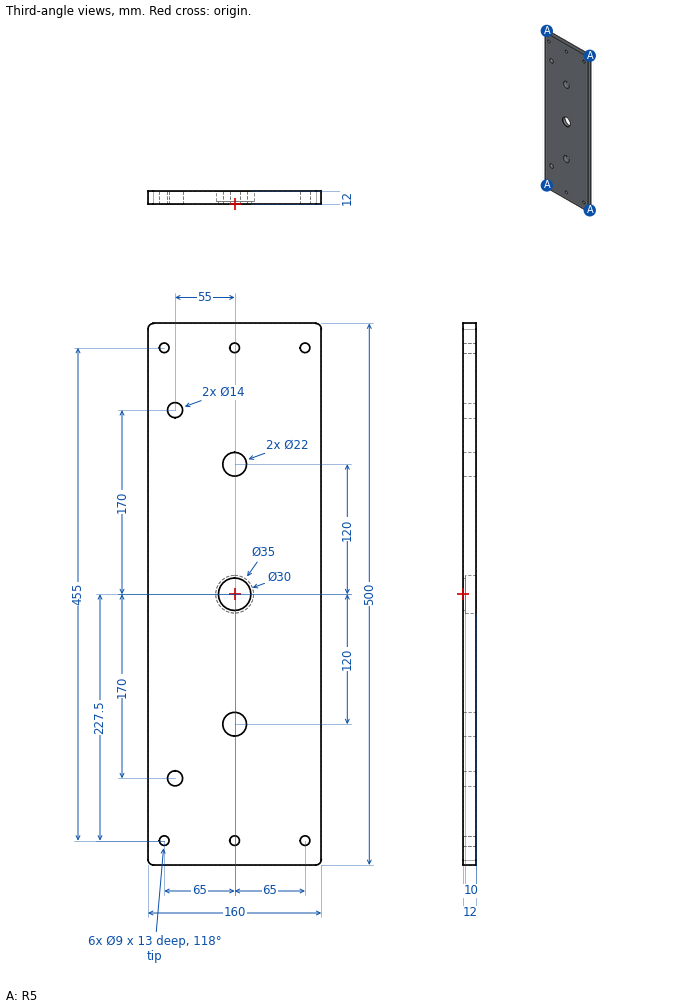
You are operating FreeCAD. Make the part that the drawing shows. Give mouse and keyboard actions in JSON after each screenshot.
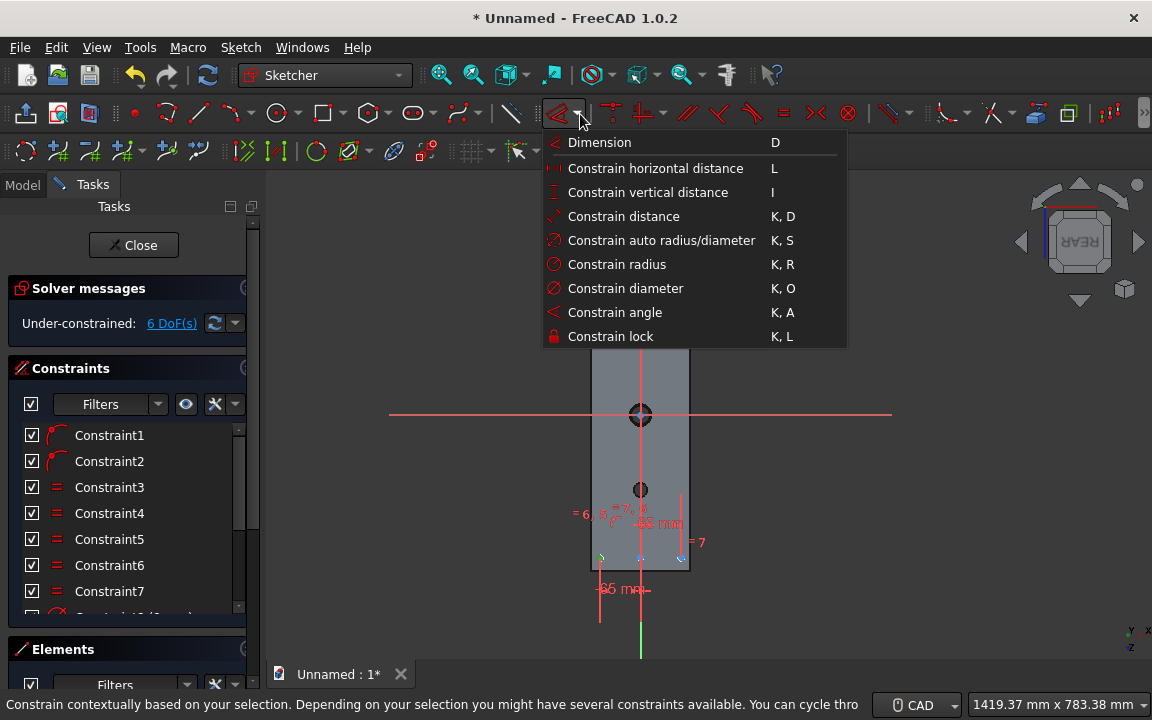
{"action": "left_click", "coordinate": [695, 192]}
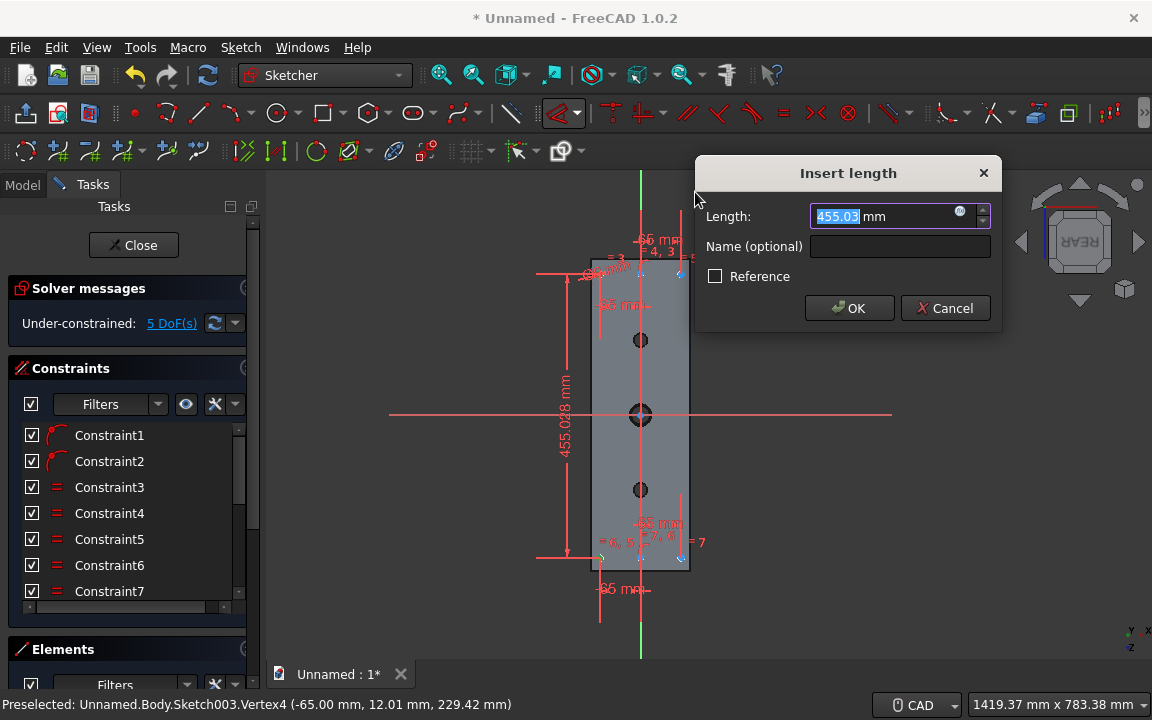
{"action": "type", "text": "455"}
{"action": "key", "text": "Return"}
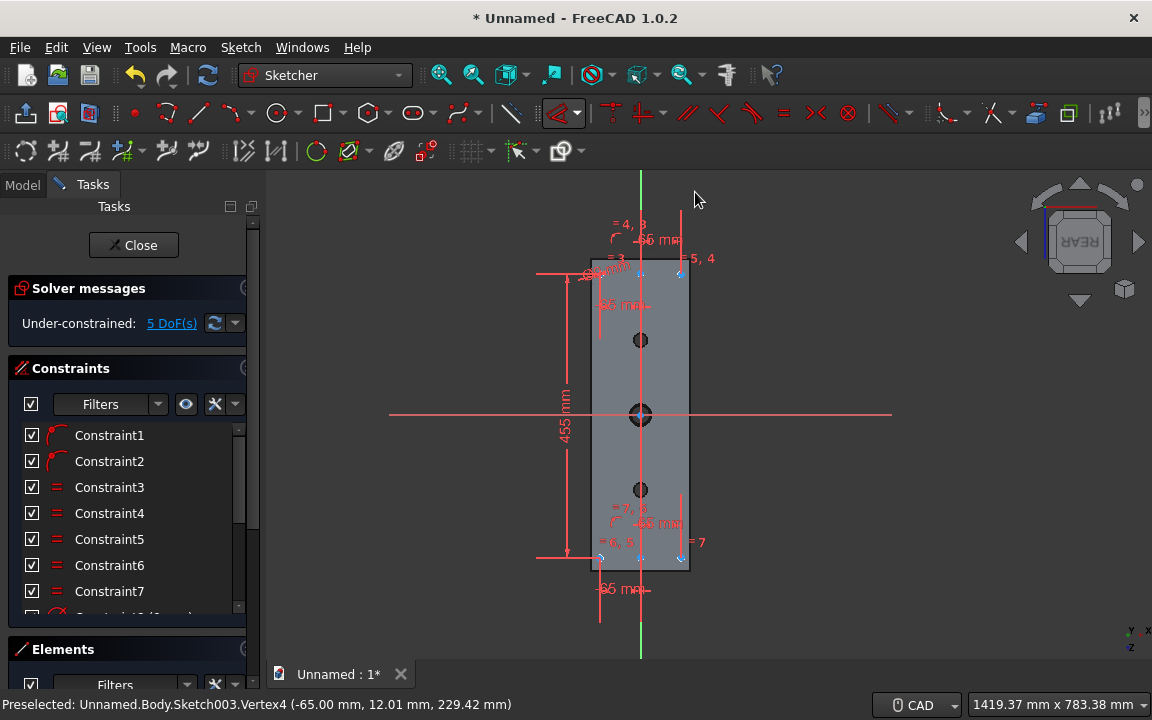
{"action": "left_click", "coordinate": [641, 274]}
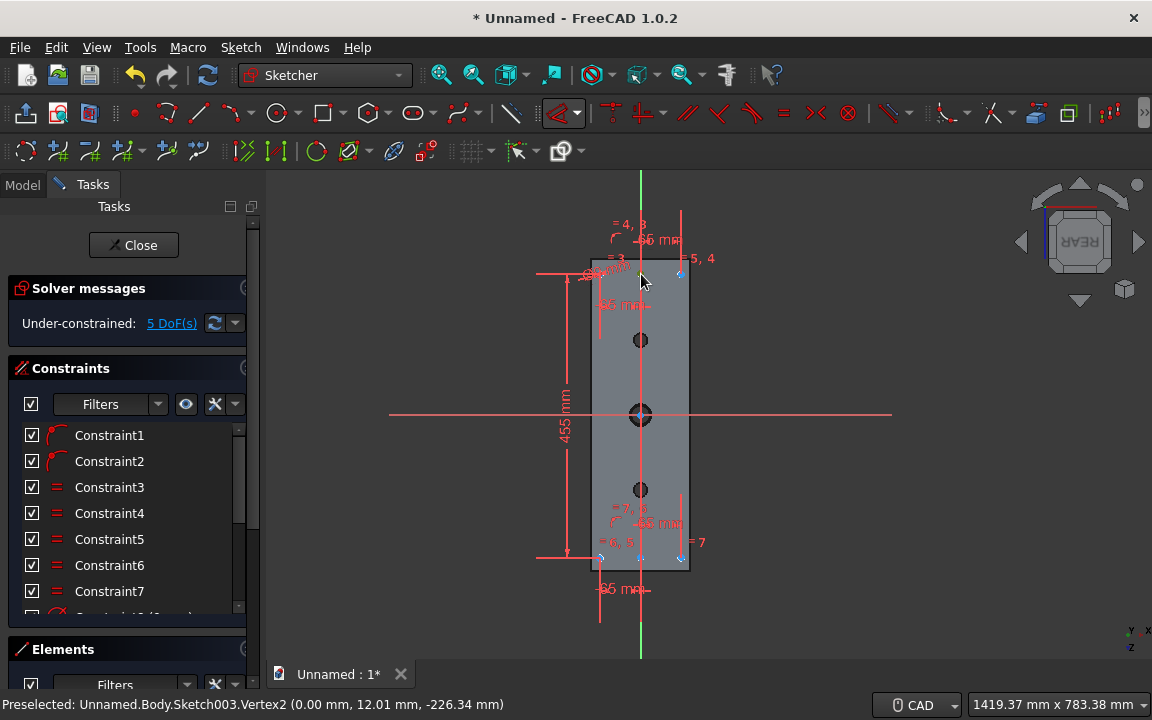
{"action": "left_click", "coordinate": [600, 558]}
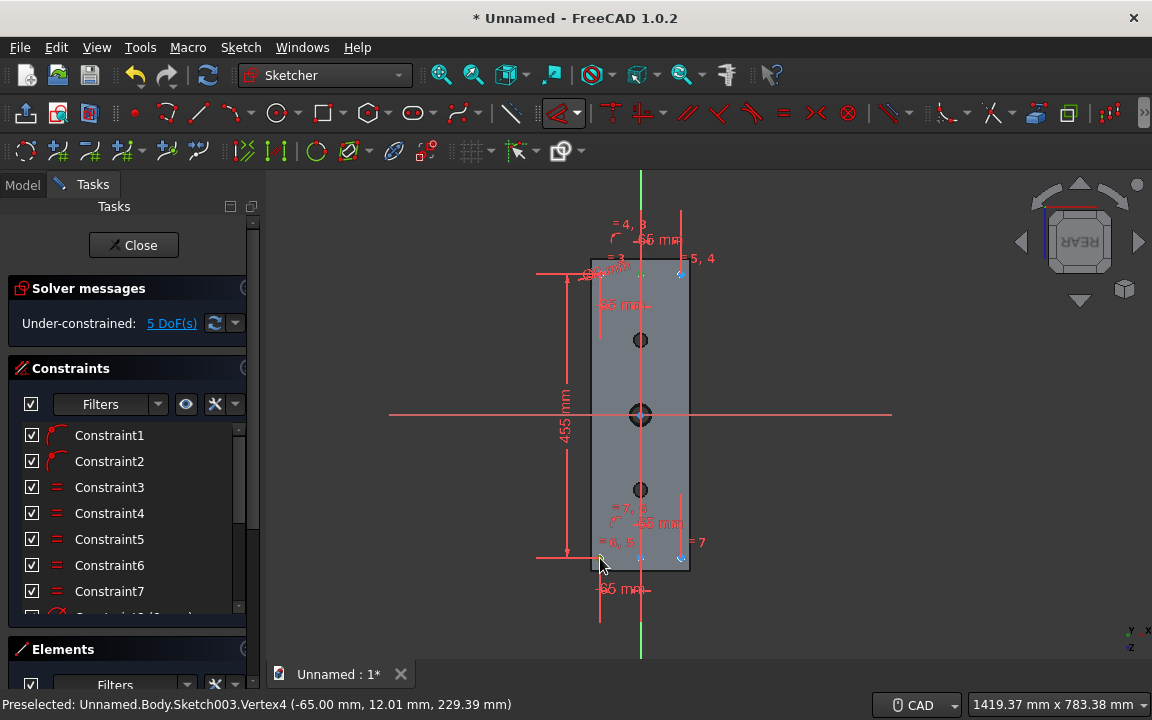
{"action": "key", "text": "i"}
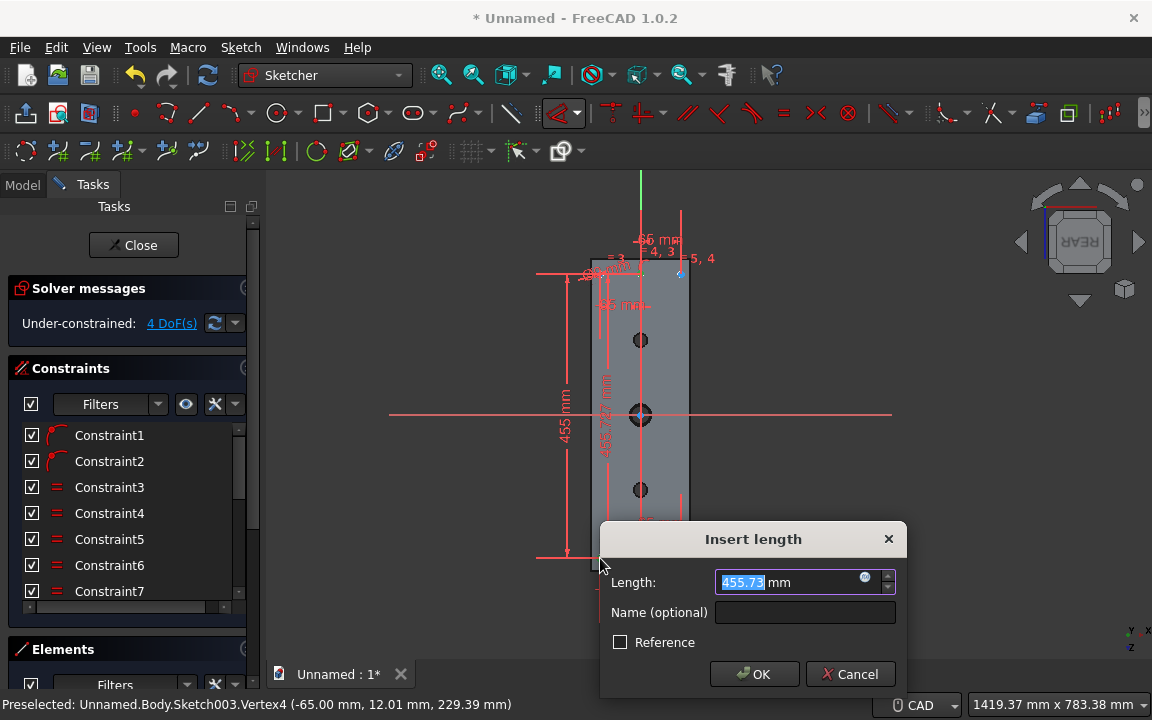
{"action": "type", "text": "455"}
{"action": "key", "text": "Return"}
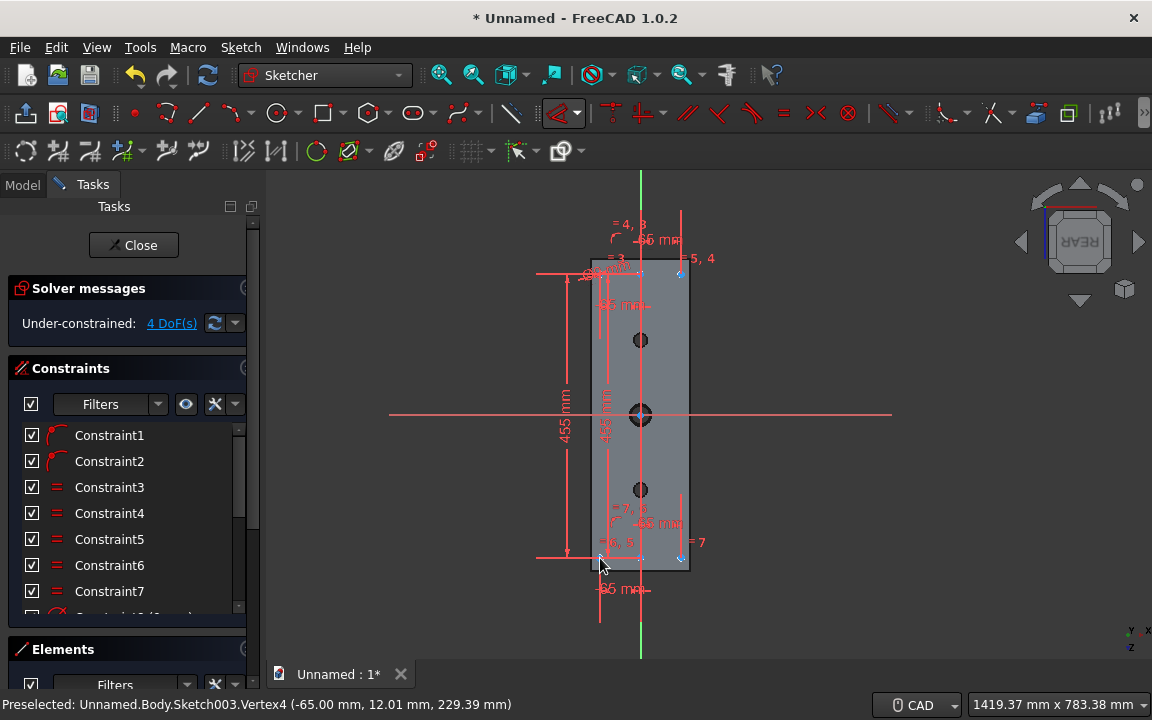
{"action": "left_click", "coordinate": [681, 274]}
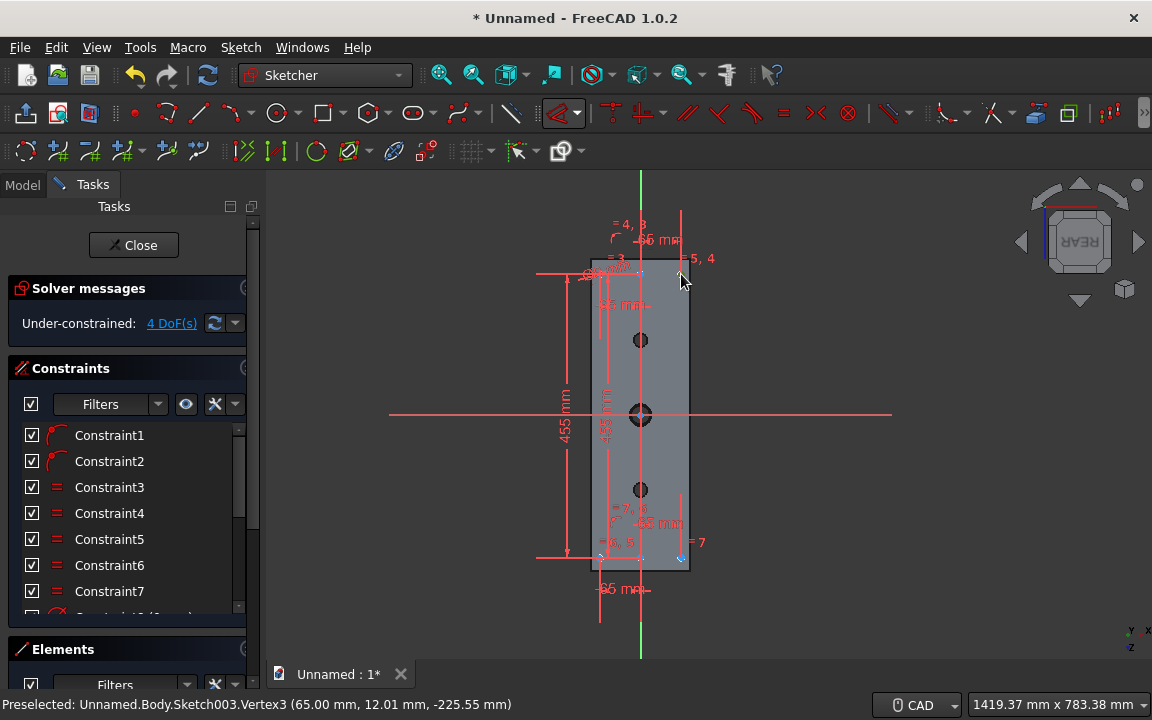
{"action": "left_click", "coordinate": [600, 558]}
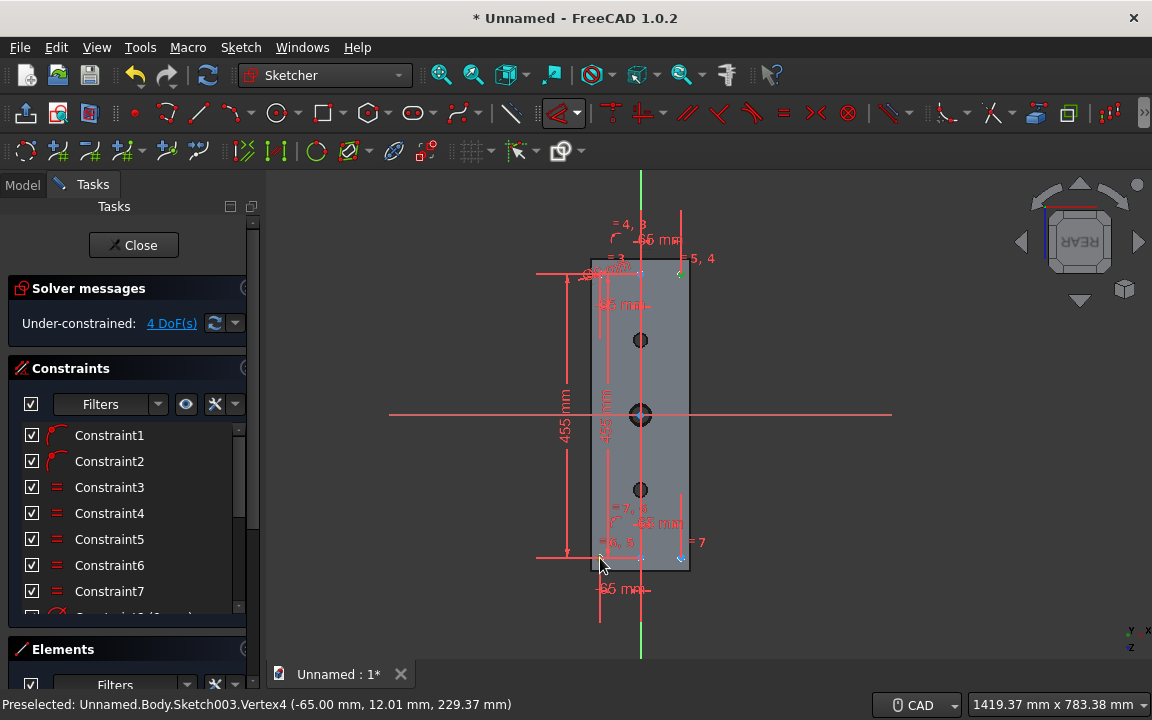
{"action": "left_click", "coordinate": [580, 114]}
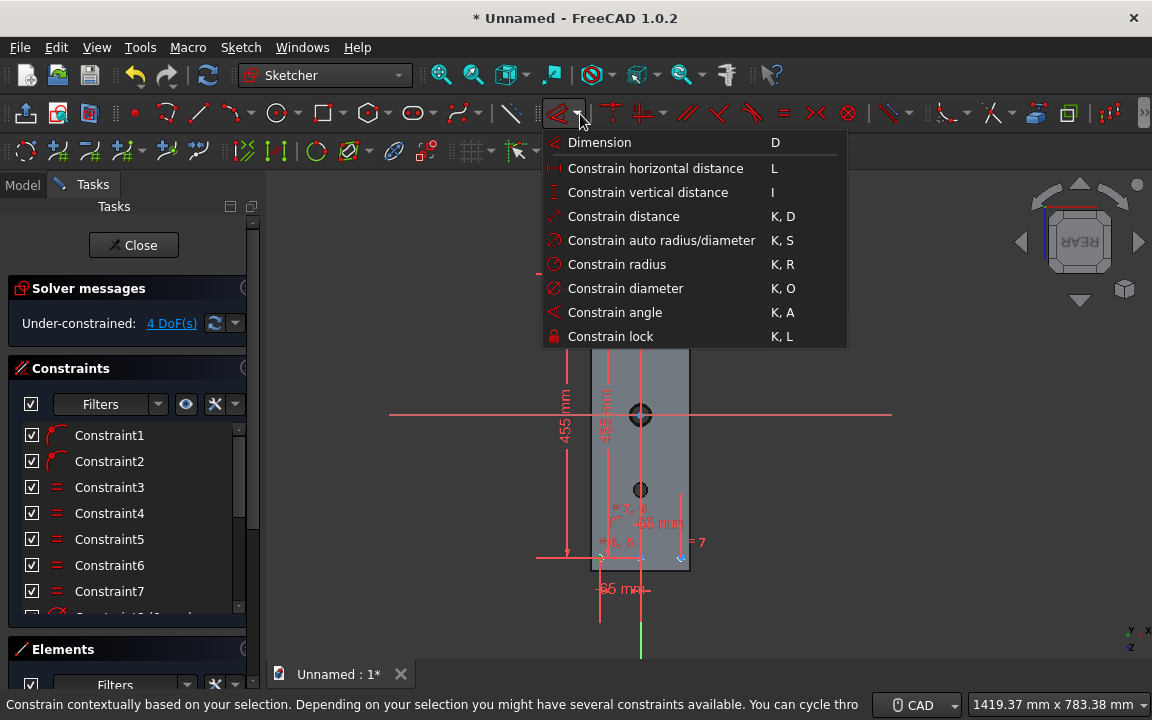
{"action": "left_click", "coordinate": [695, 192]}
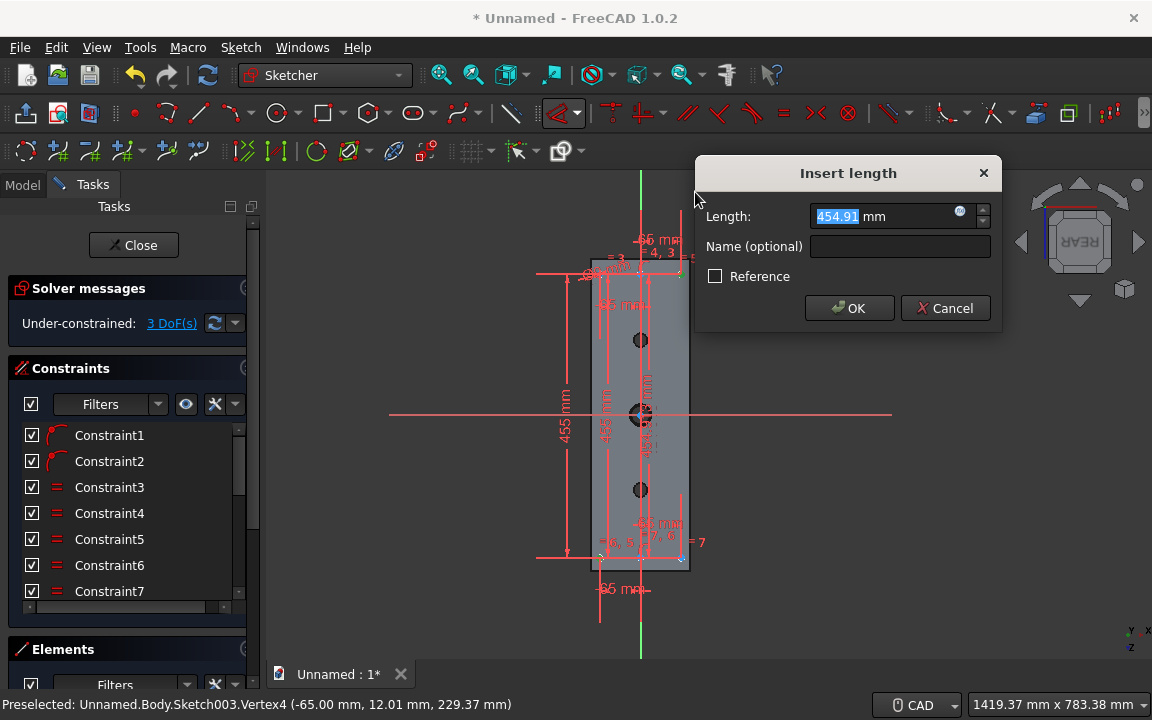
{"action": "type", "text": "455"}
{"action": "key", "text": "Return"}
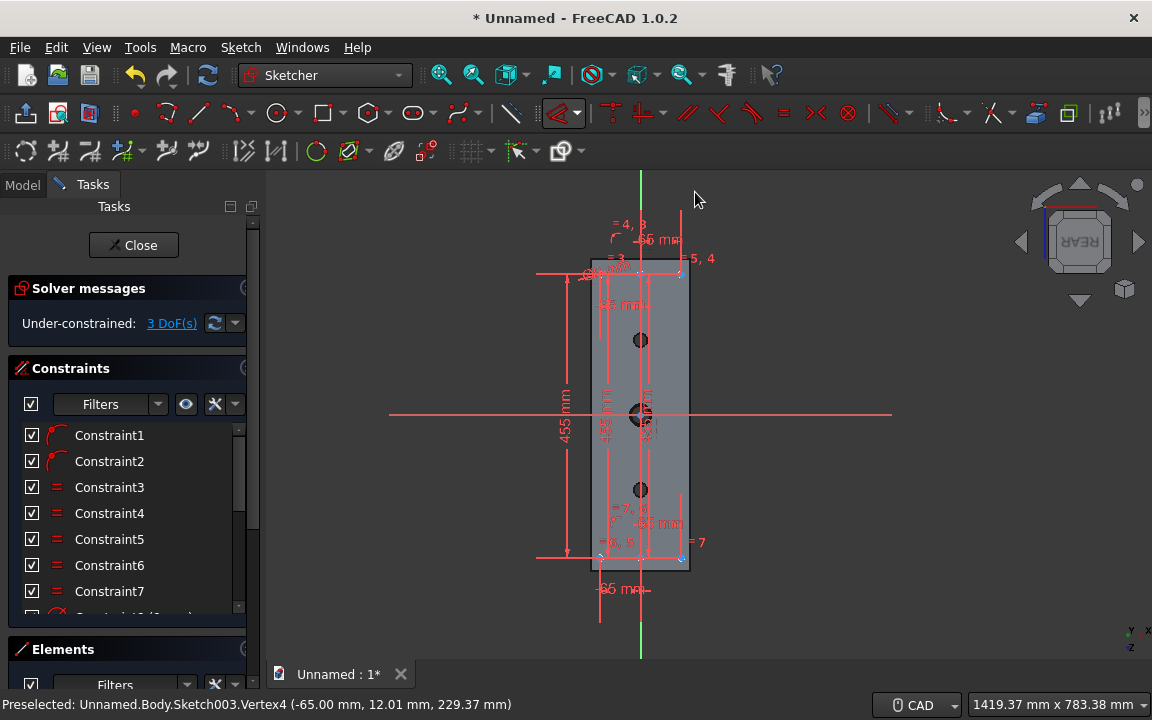
{"action": "left_click", "coordinate": [641, 274]}